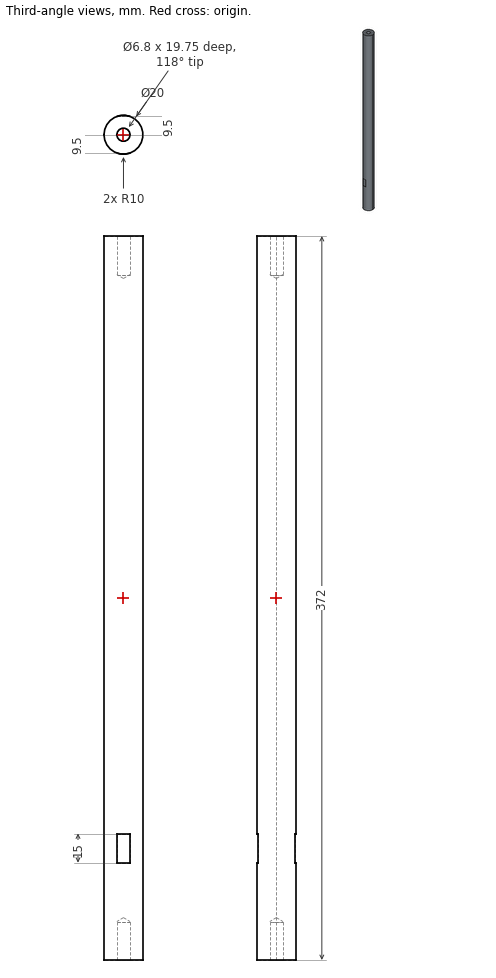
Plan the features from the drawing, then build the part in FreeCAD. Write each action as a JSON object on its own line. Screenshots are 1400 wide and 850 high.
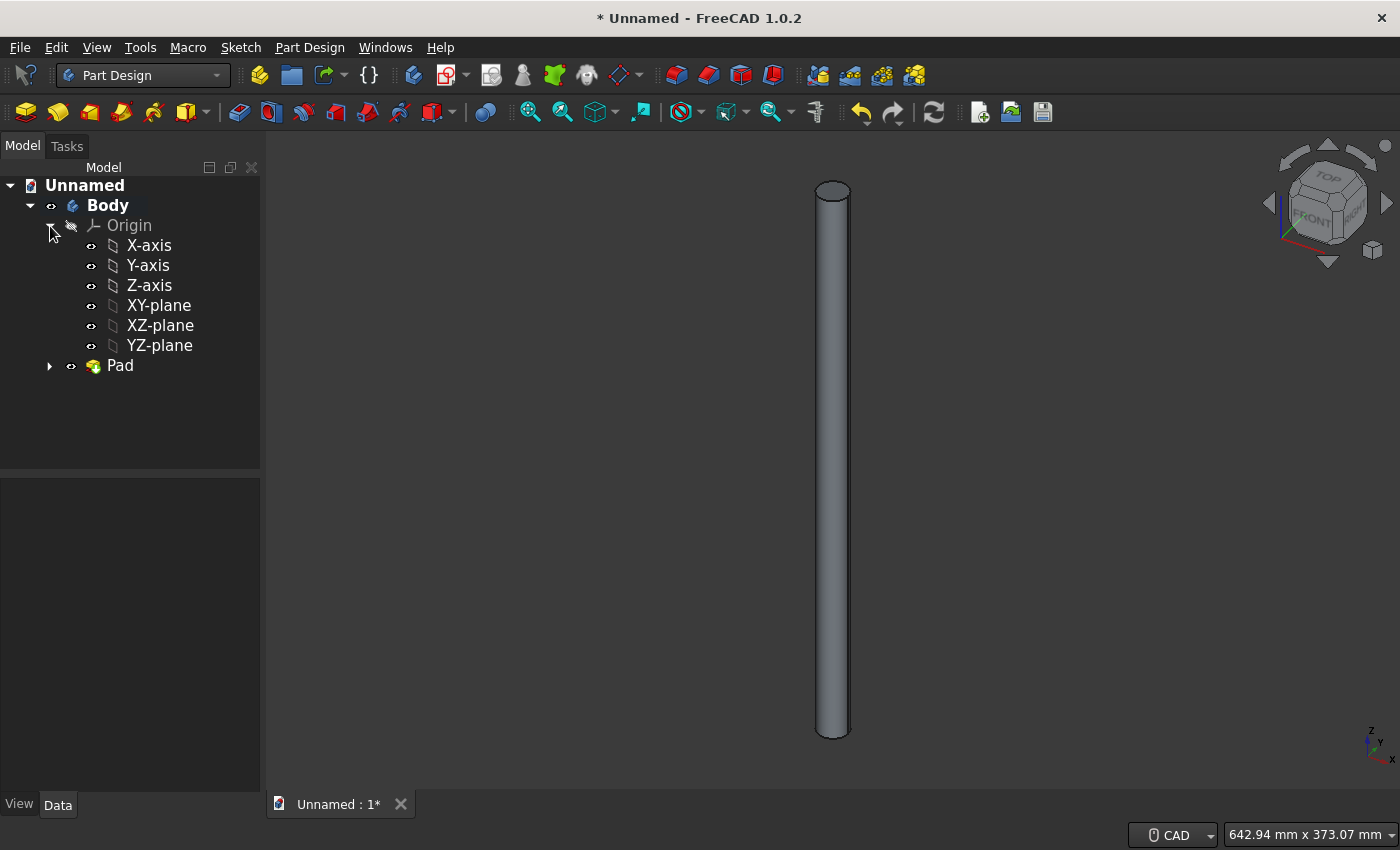
{"action": "left_click", "coordinate": [136, 306]}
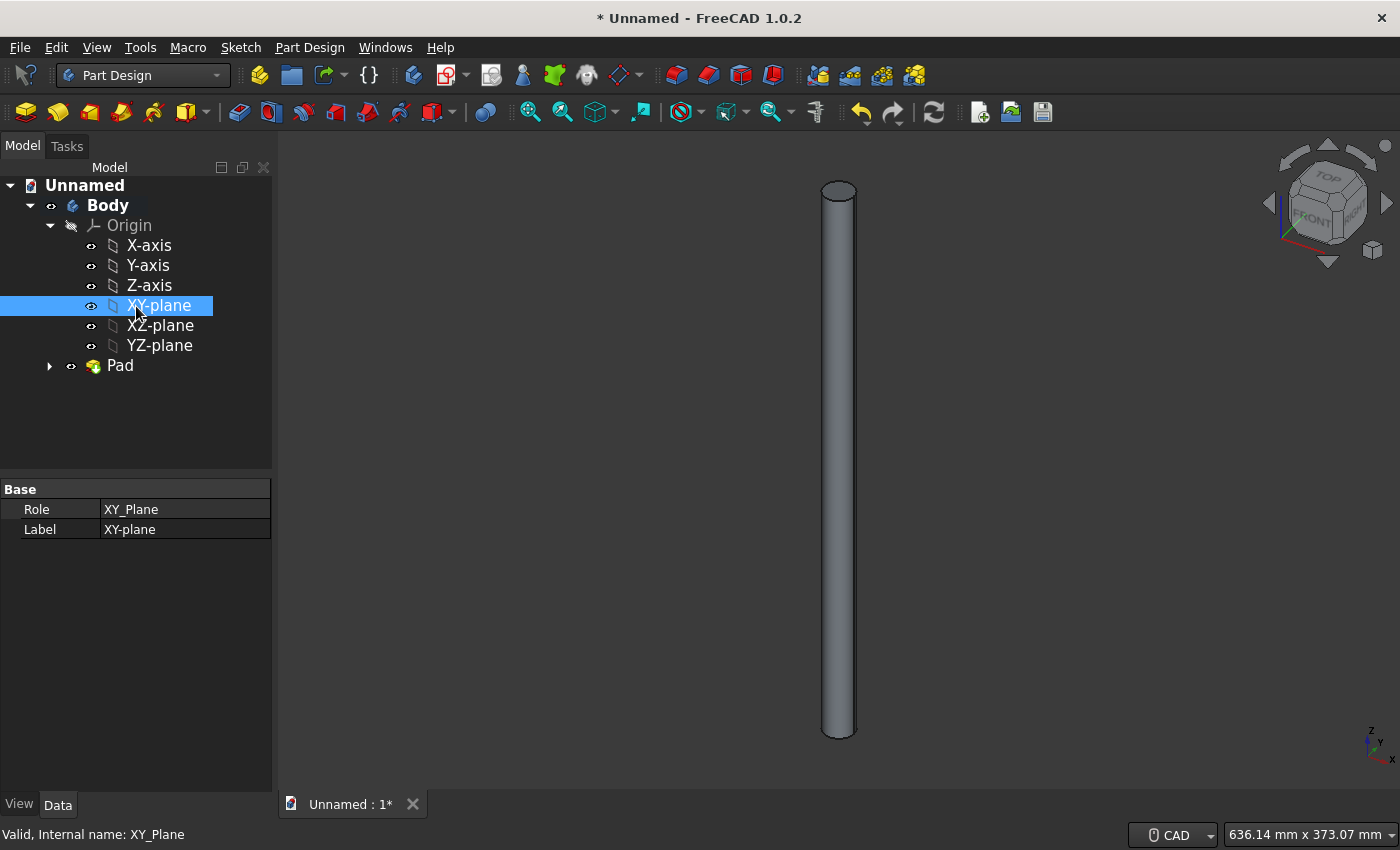
{"action": "left_click", "coordinate": [620, 76]}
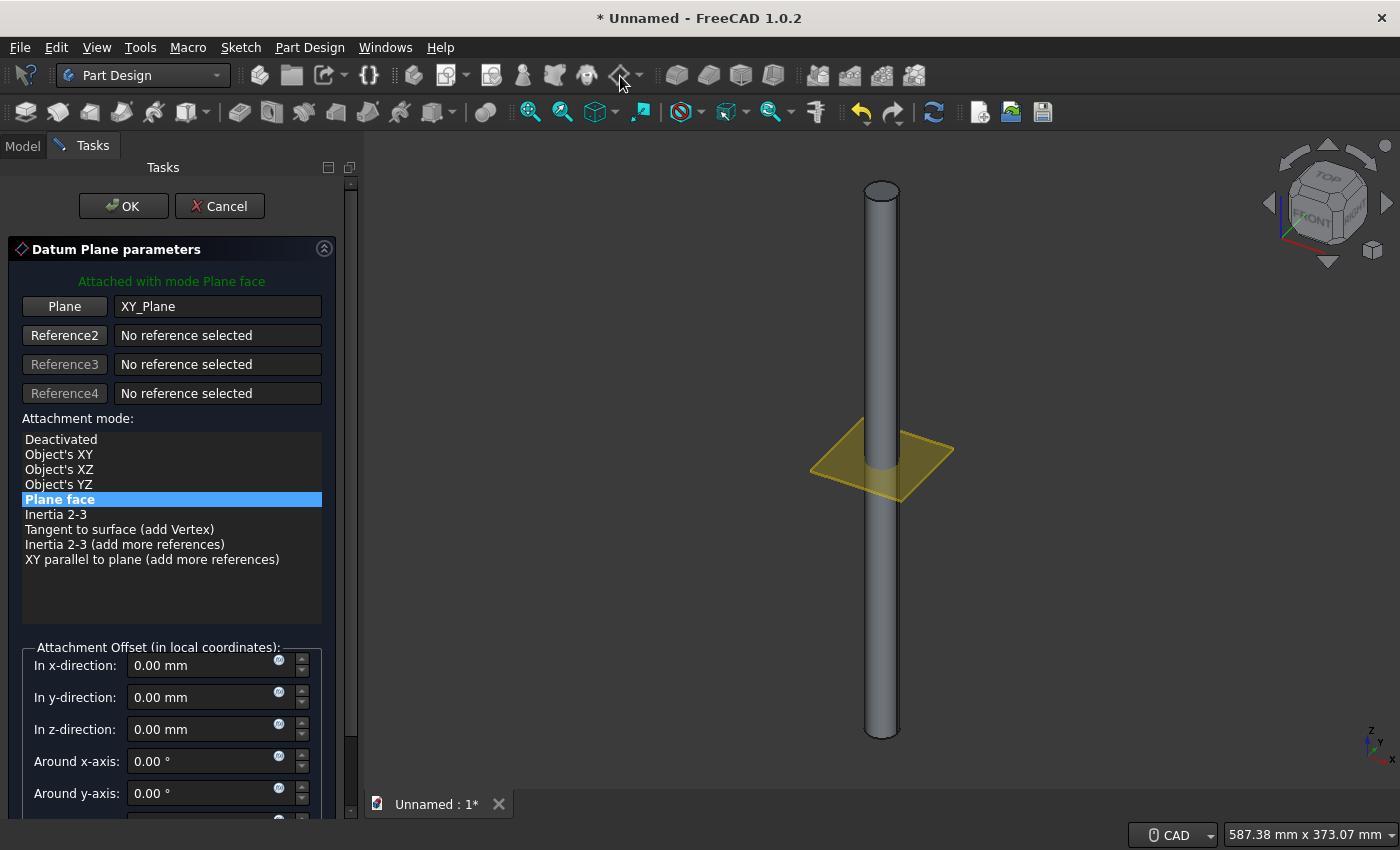
{"action": "triple_click", "coordinate": [210, 729]}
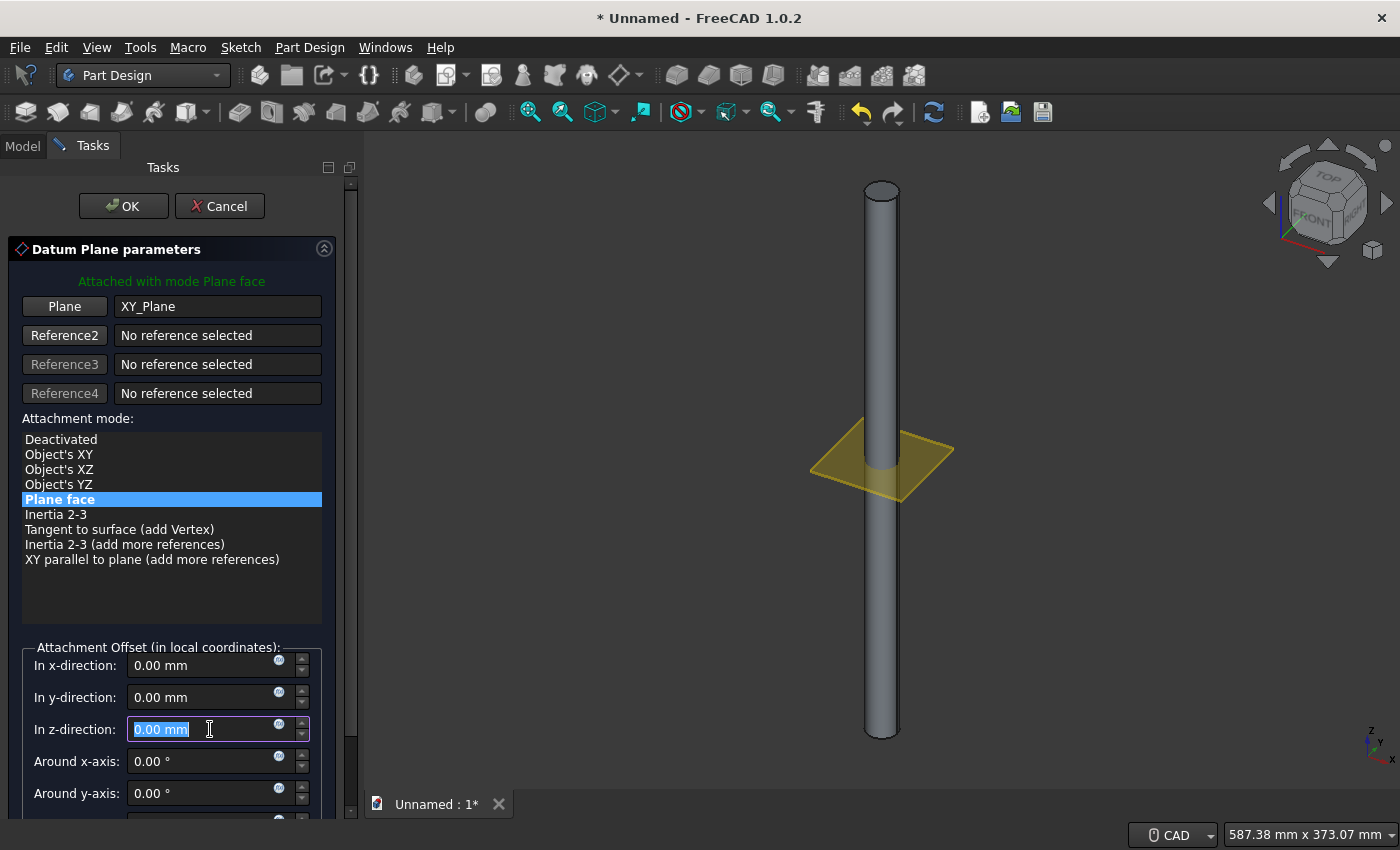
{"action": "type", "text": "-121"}
{"action": "key", "text": "Tab"}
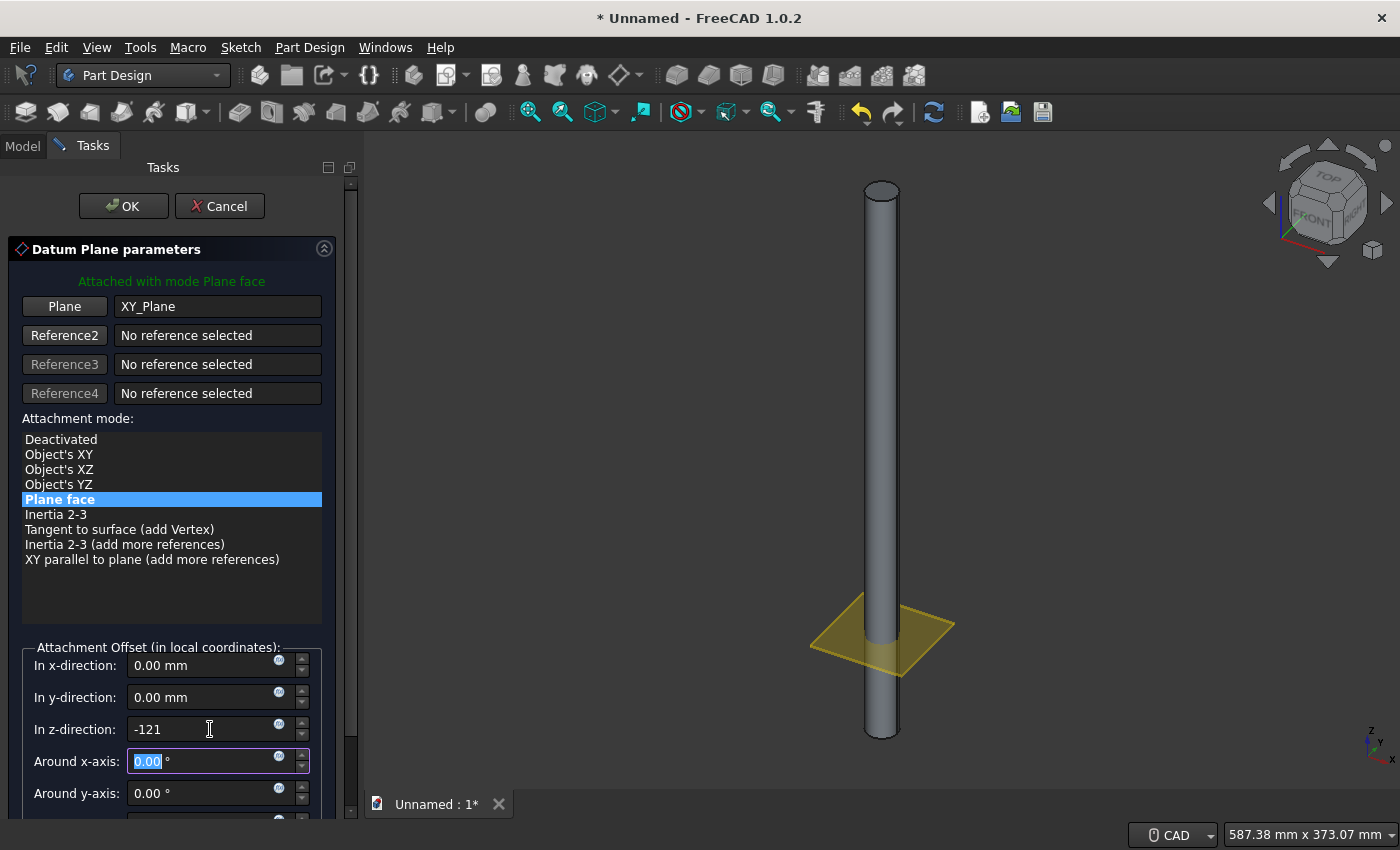
{"action": "left_click", "coordinate": [124, 206]}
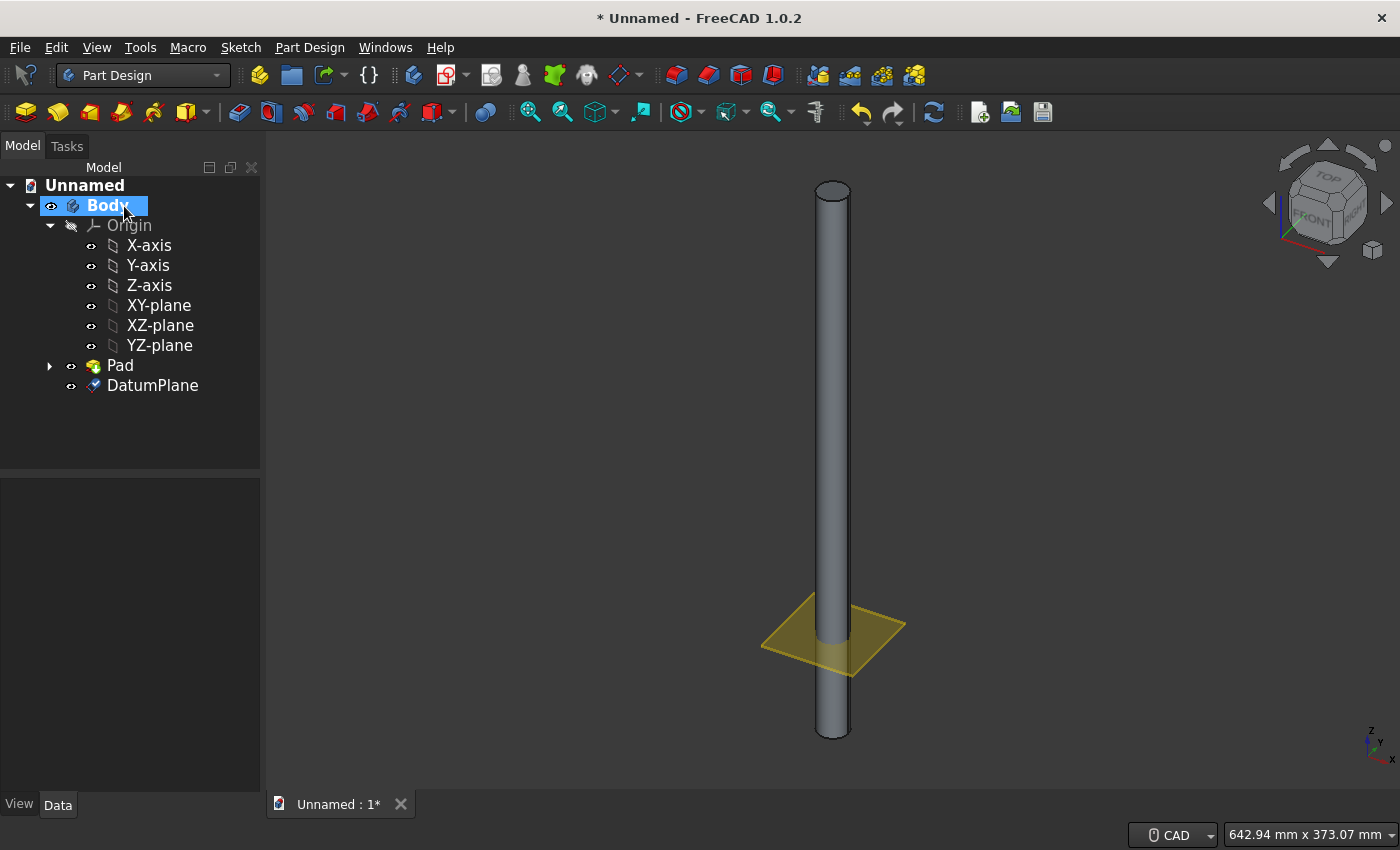
{"action": "left_click", "coordinate": [116, 386]}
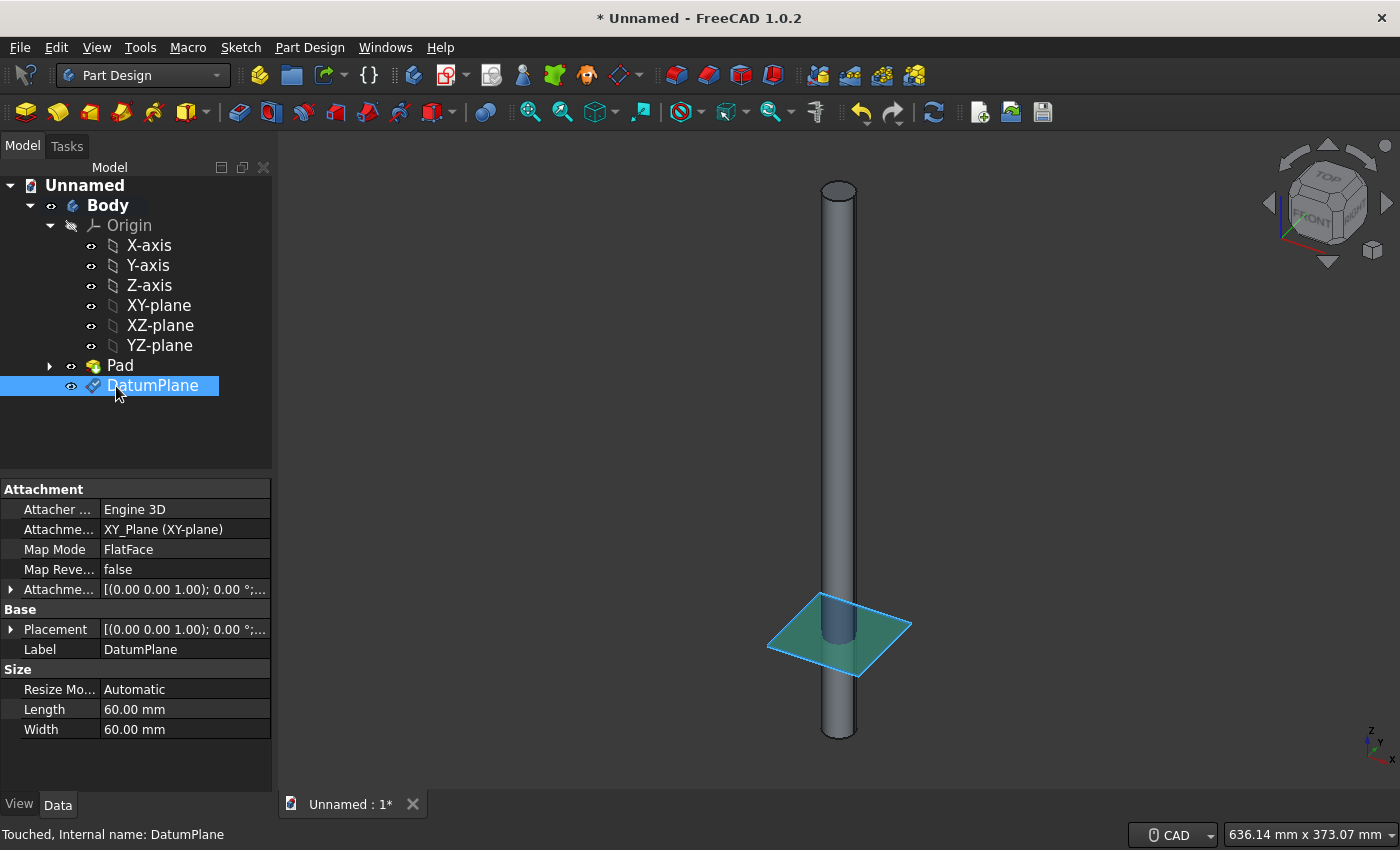
{"action": "left_click", "coordinate": [446, 76]}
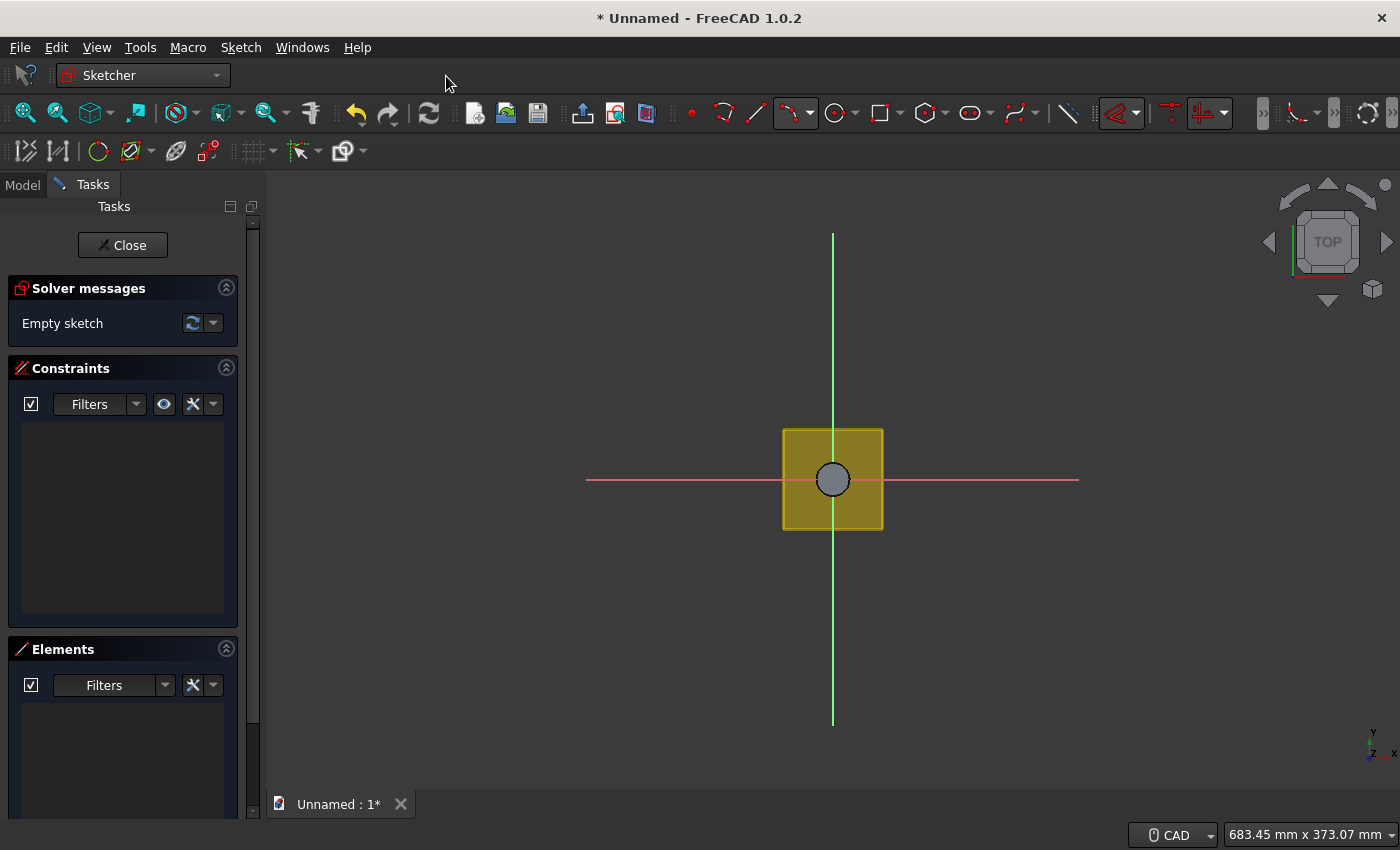
{"action": "key", "text": "q s"}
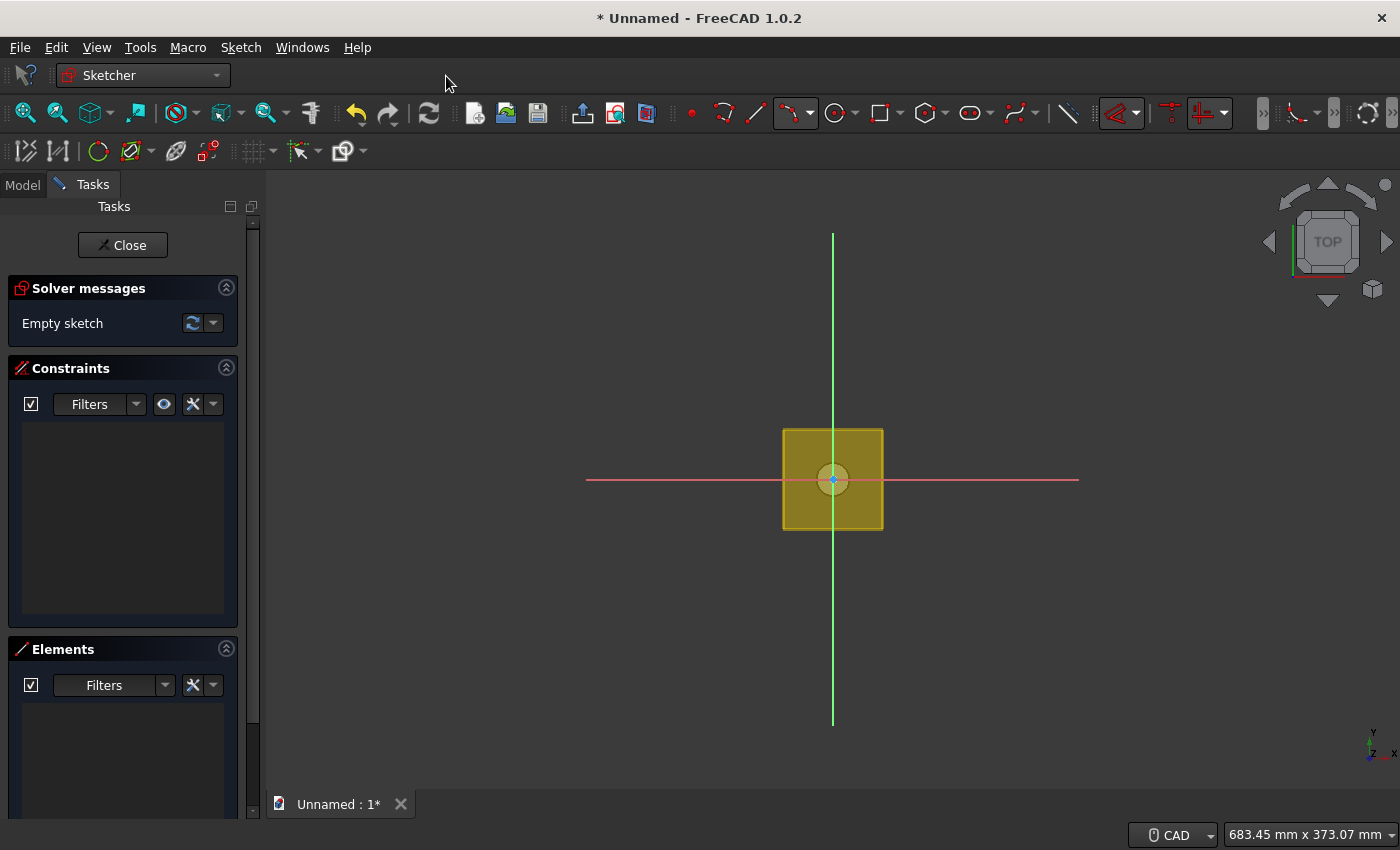
{"action": "scroll", "coordinate": [840, 480], "scroll_direction": "up", "scroll_amount": 12}